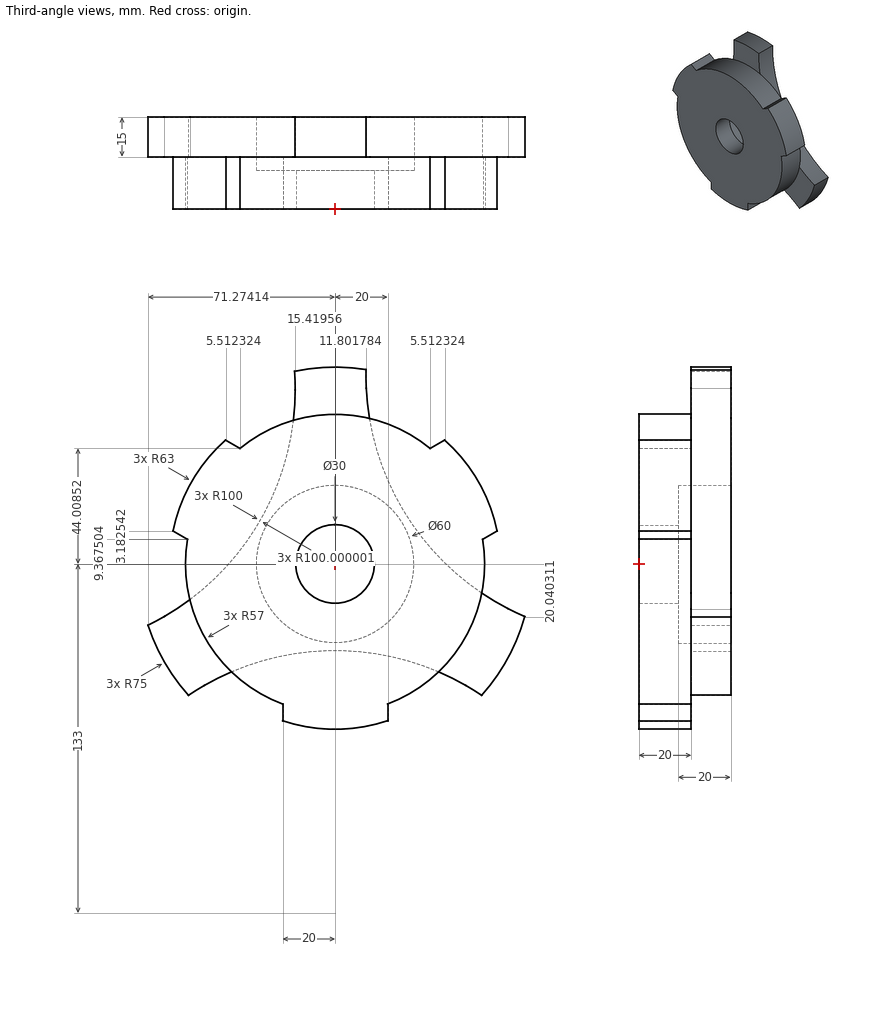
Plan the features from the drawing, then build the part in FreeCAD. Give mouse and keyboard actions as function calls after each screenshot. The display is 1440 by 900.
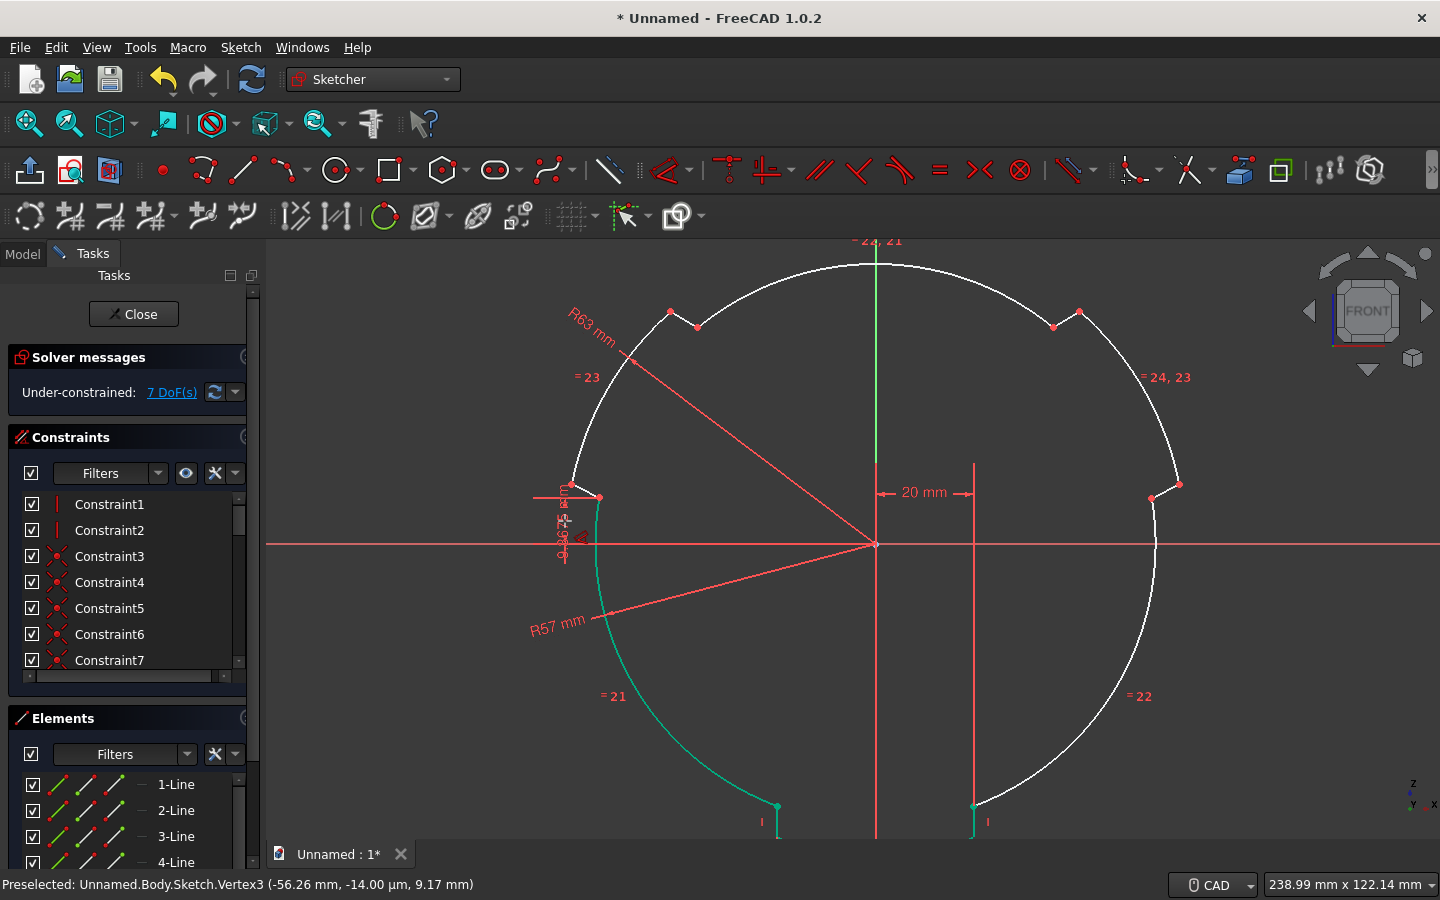
click(698, 328)
click(664, 436)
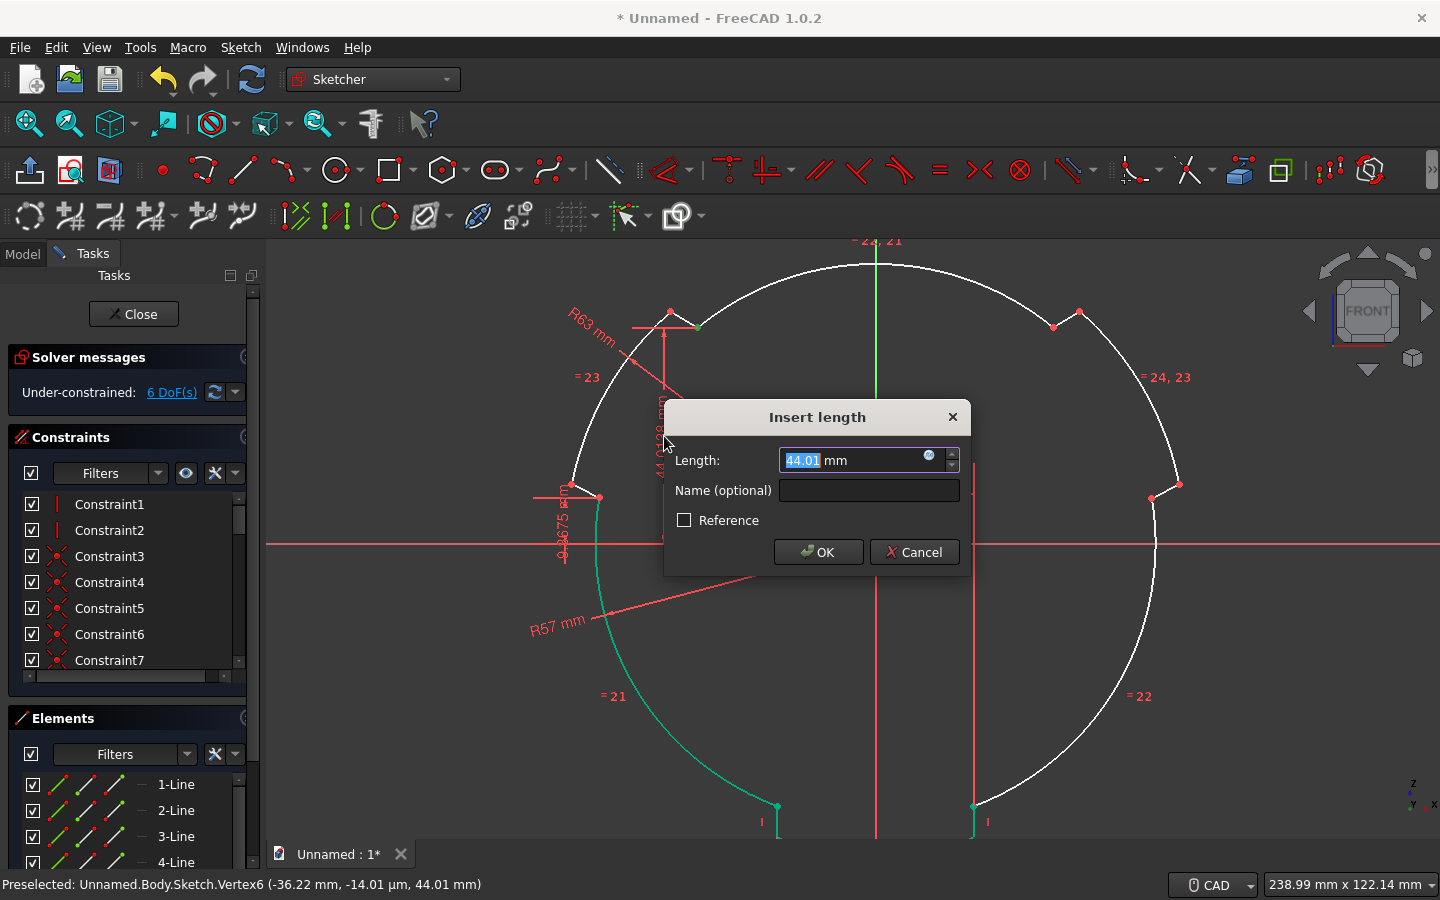
text(44.00852)
key(Return)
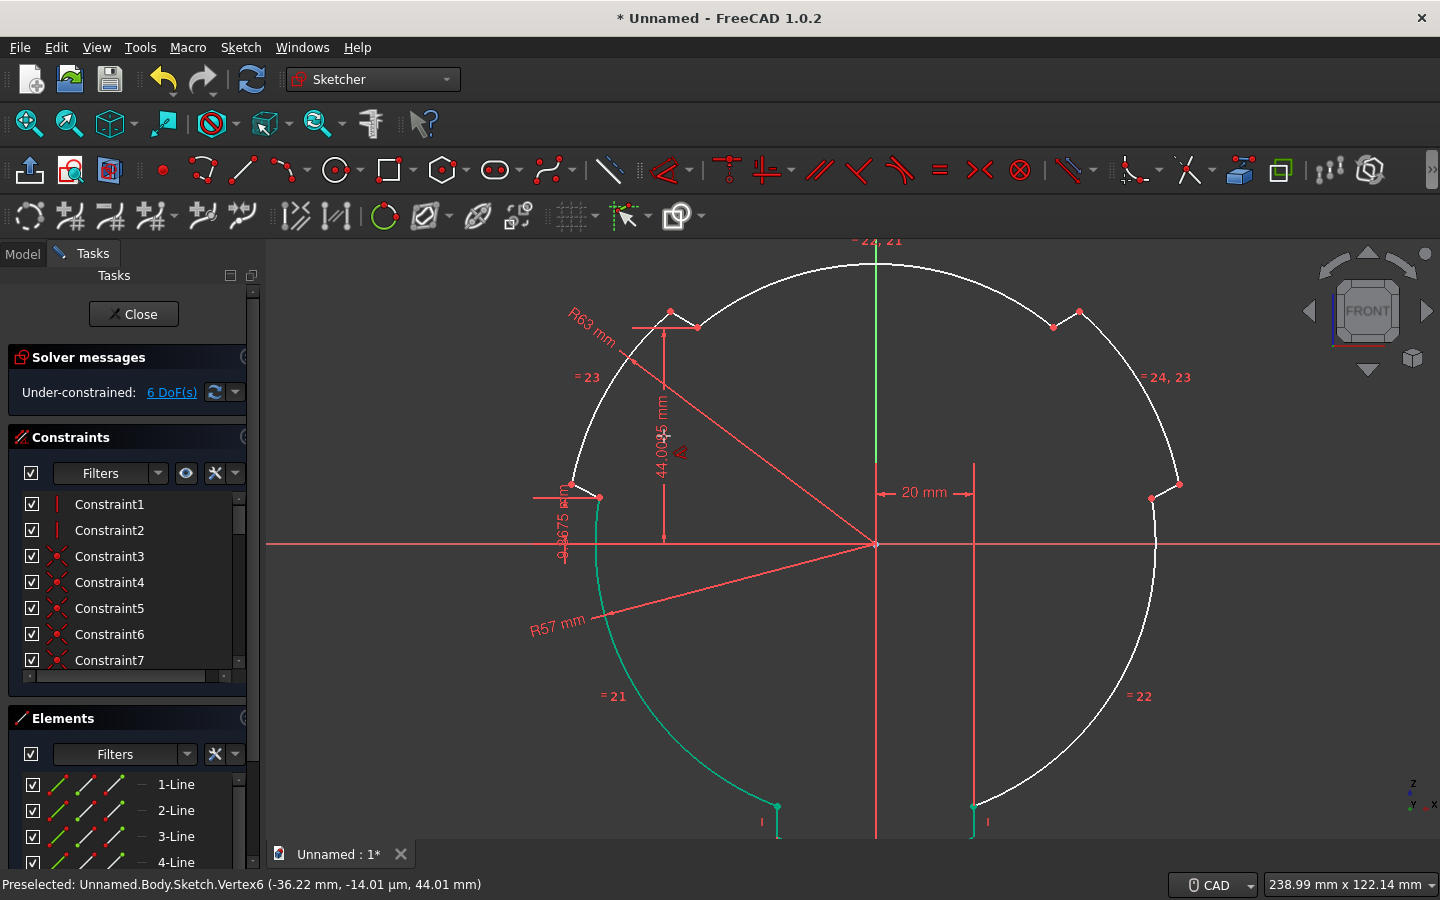
click(1053, 328)
click(1087, 436)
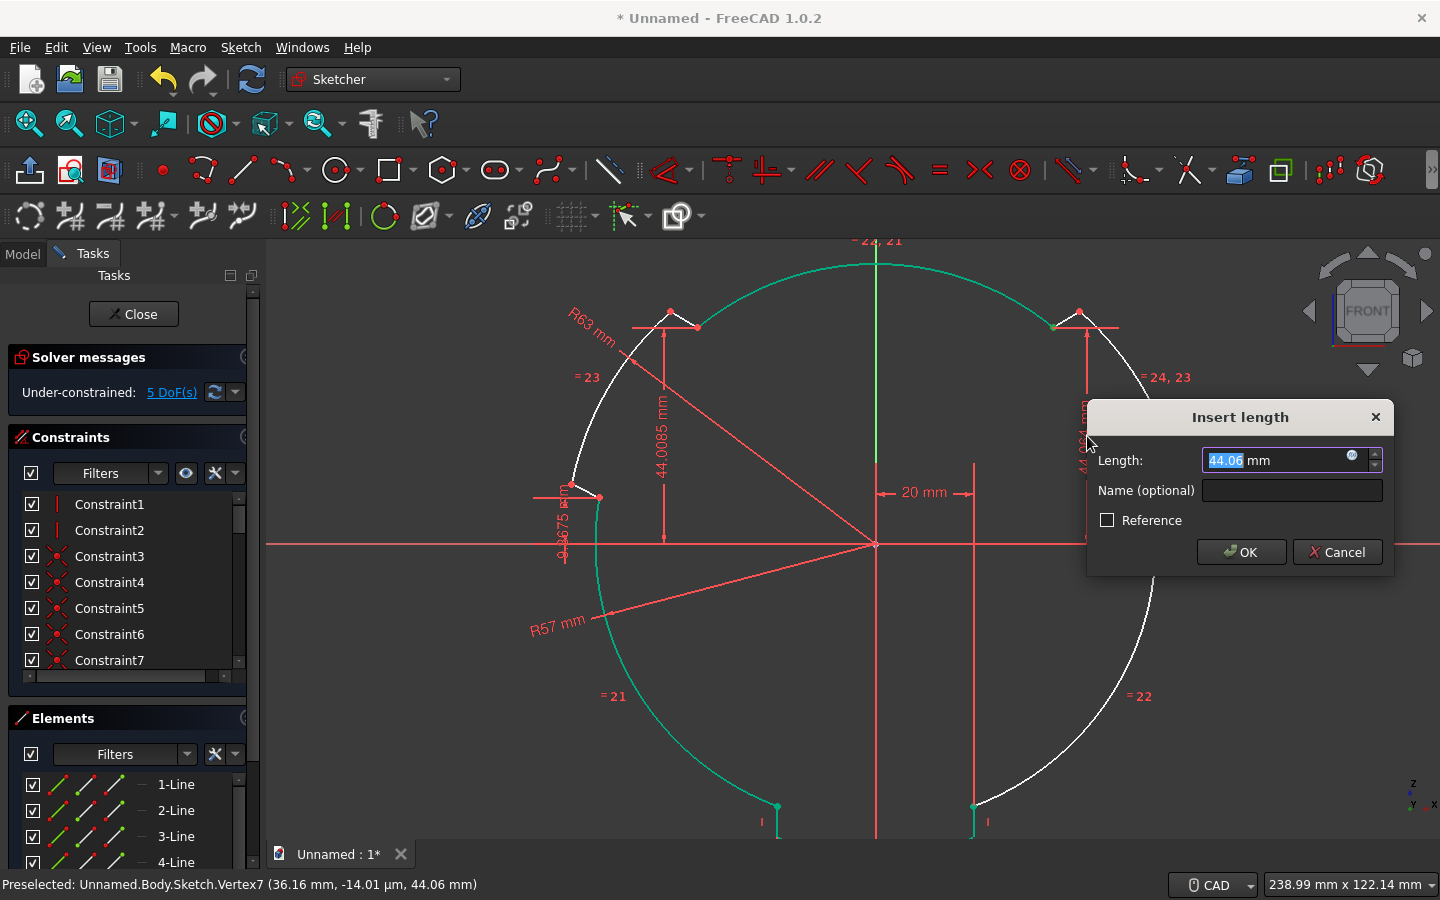
text(44.00852)
key(Return)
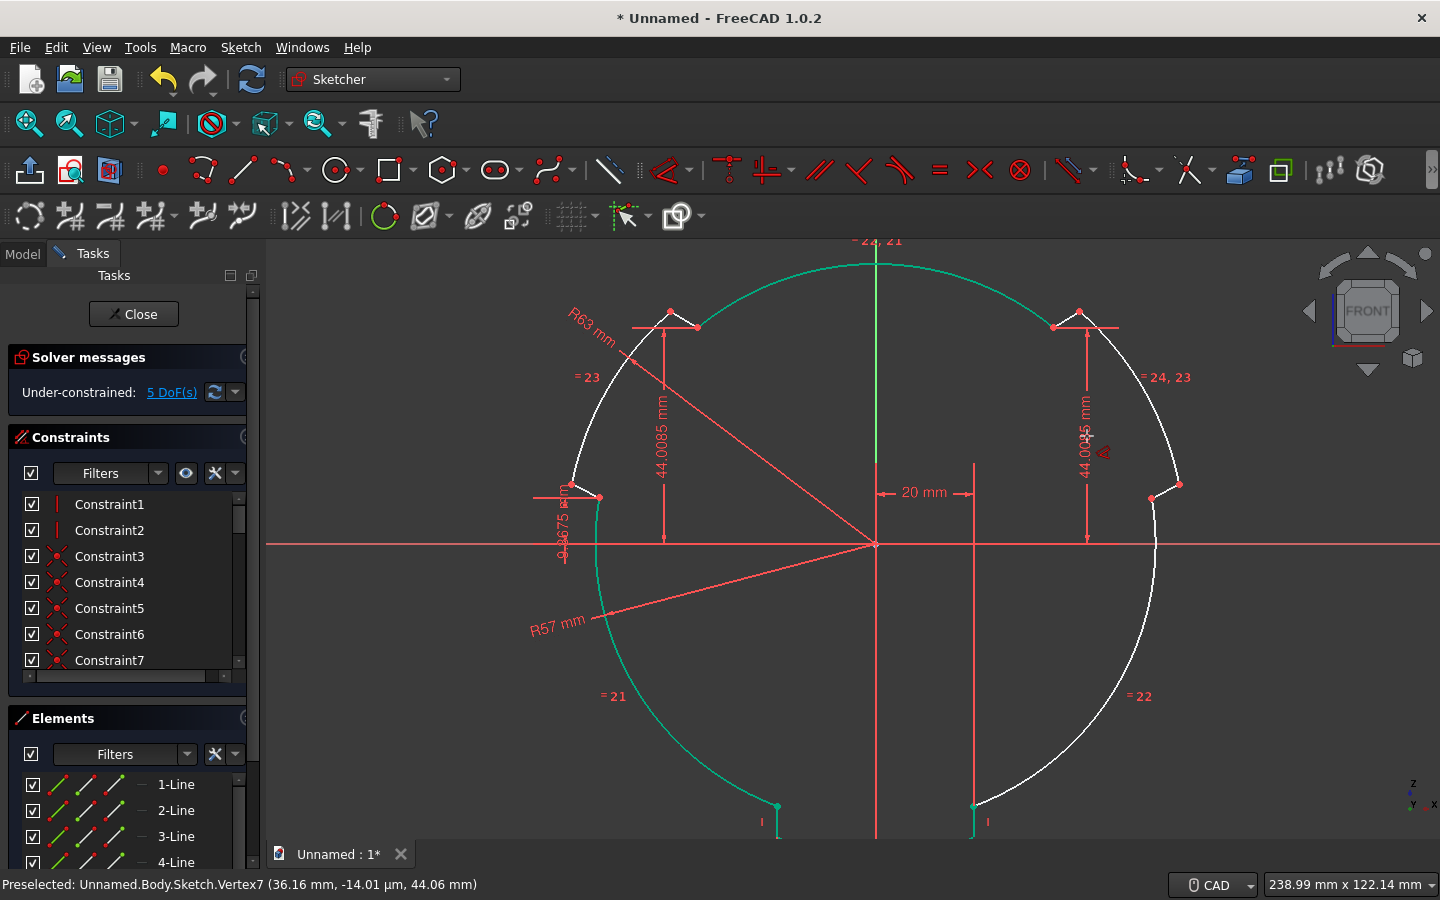
click(1152, 499)
click(1186, 521)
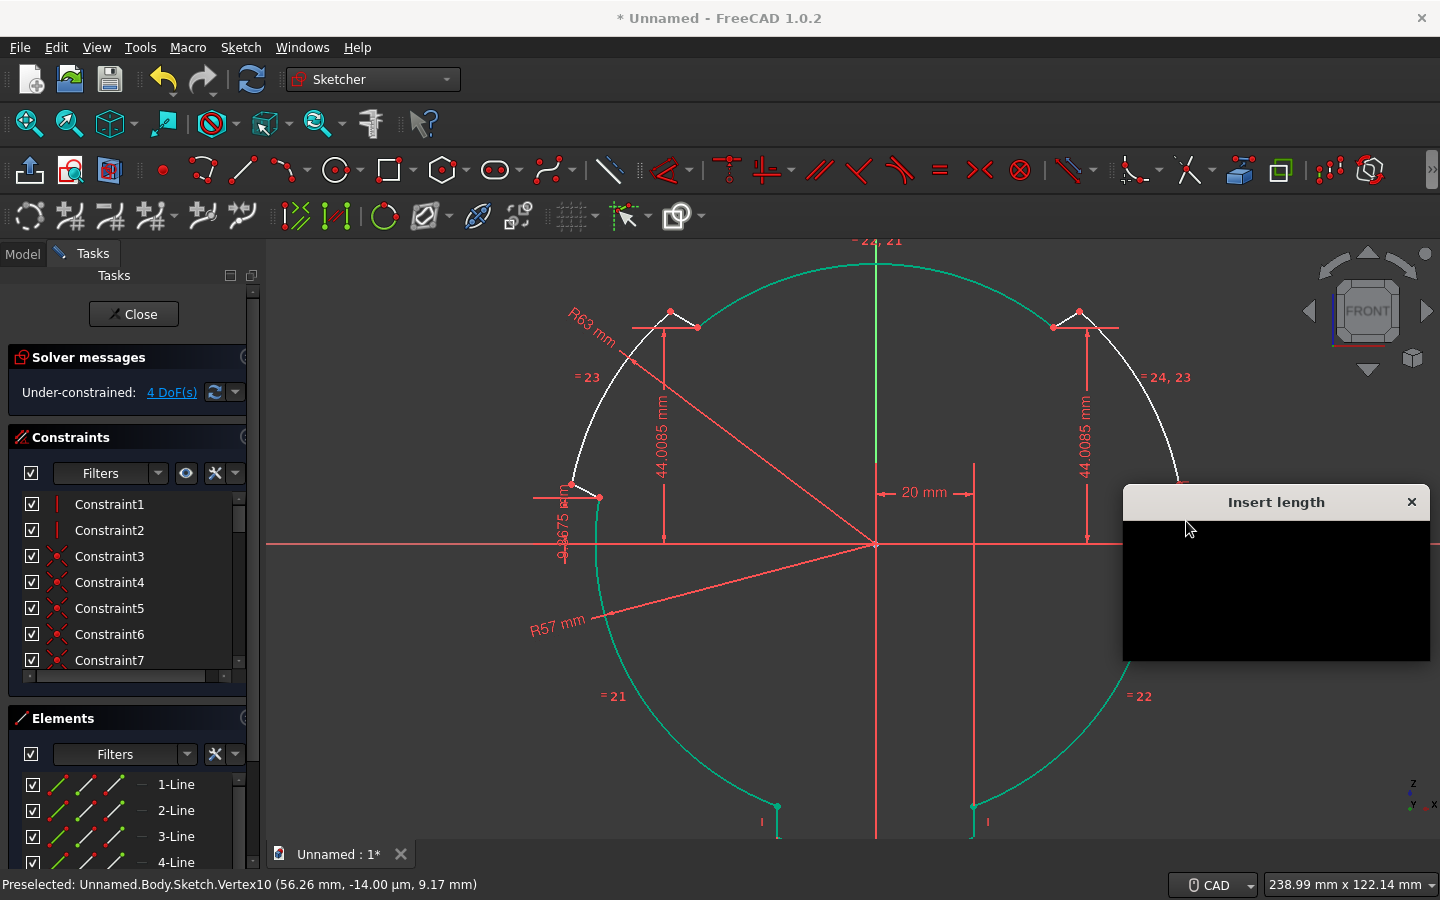
text(9.367504)
key(Return)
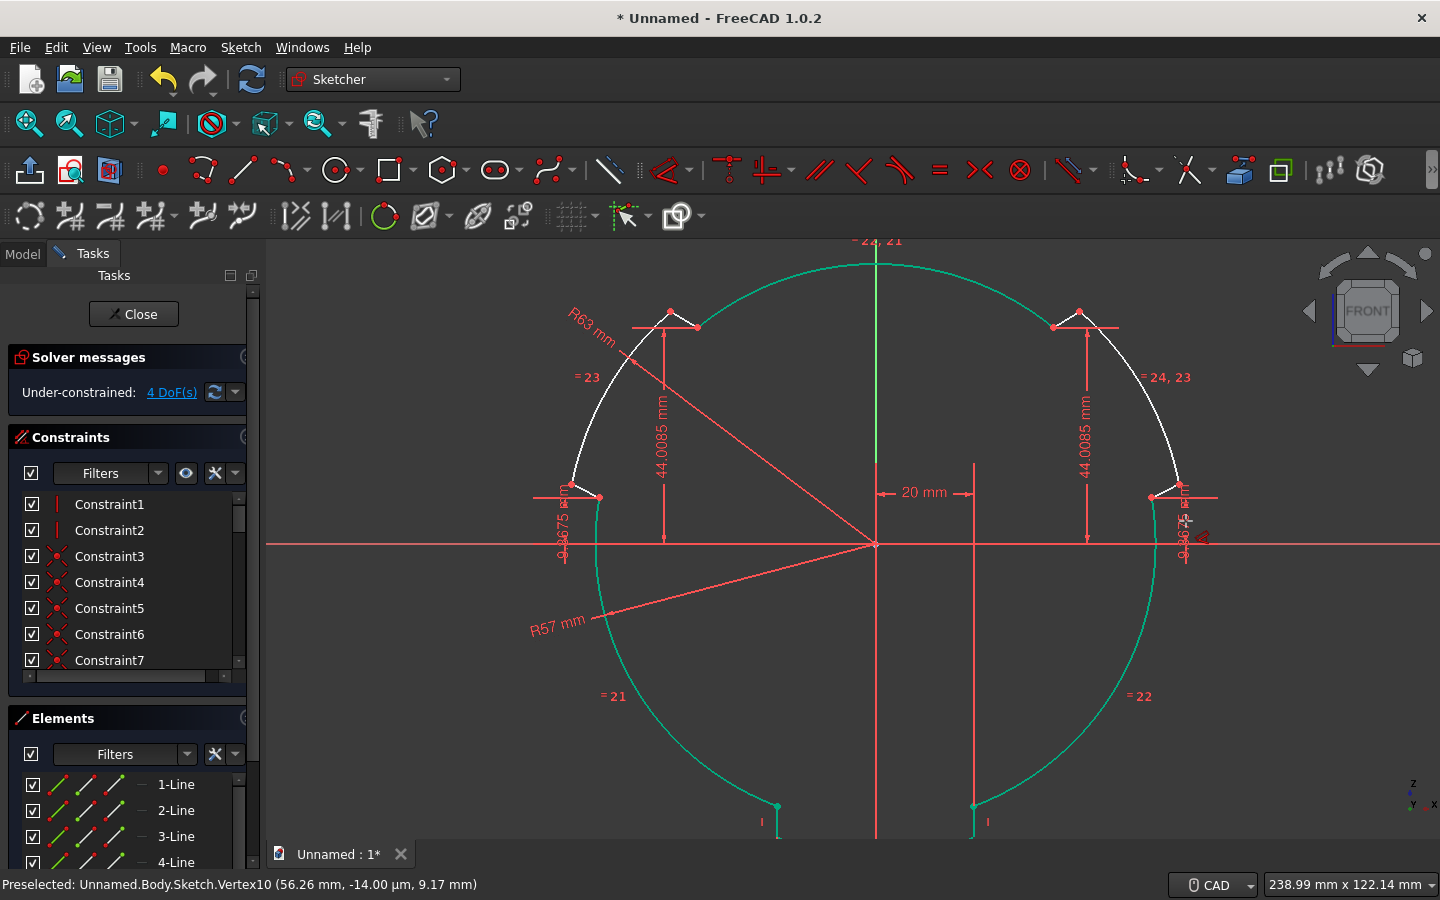
scroll(591, 494, up, 5)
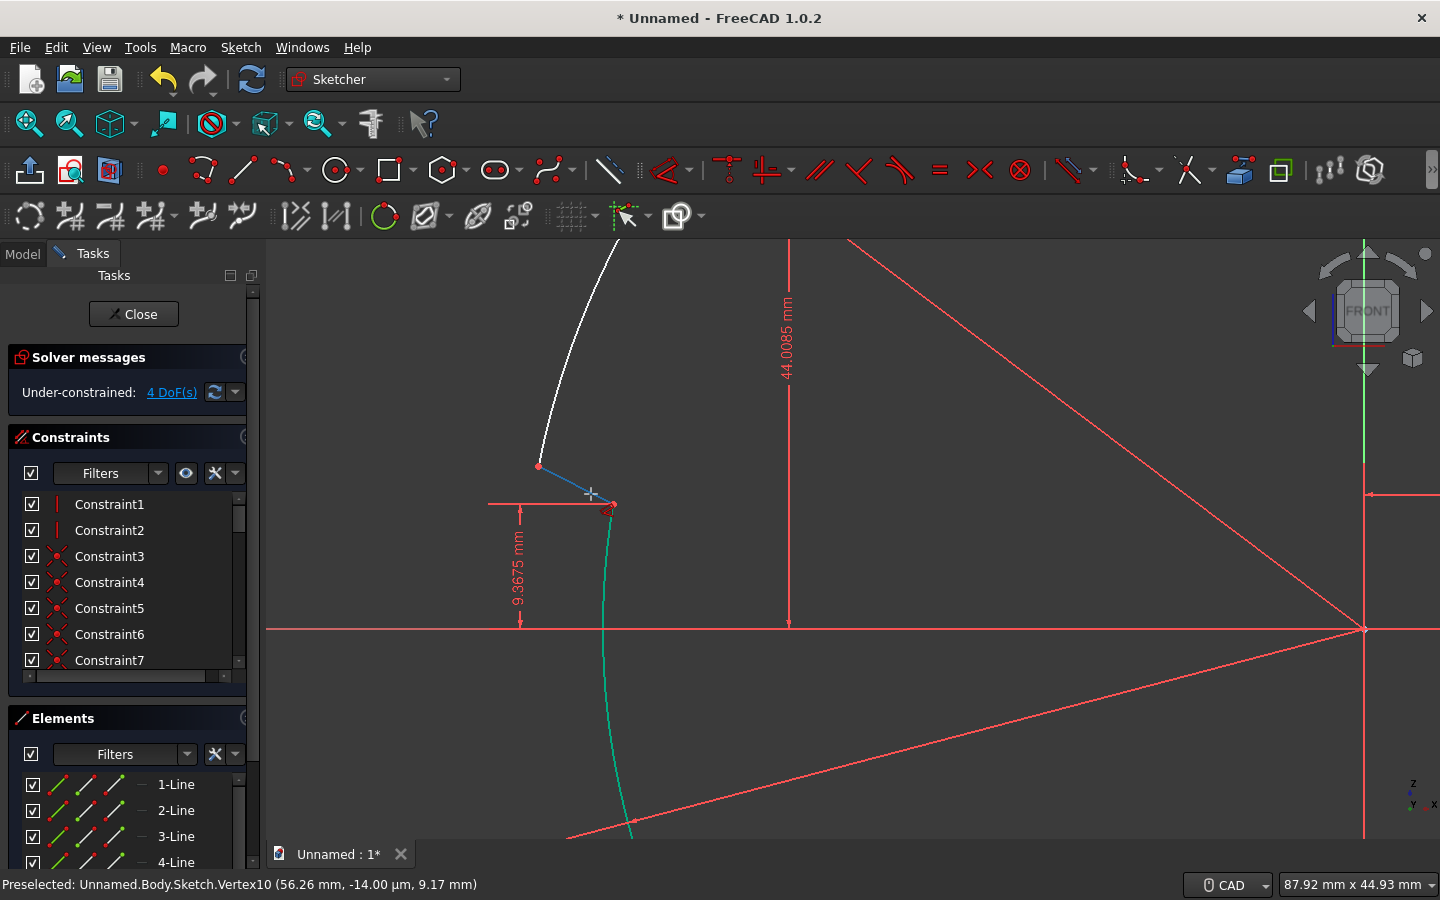
click(591, 493)
click(505, 485)